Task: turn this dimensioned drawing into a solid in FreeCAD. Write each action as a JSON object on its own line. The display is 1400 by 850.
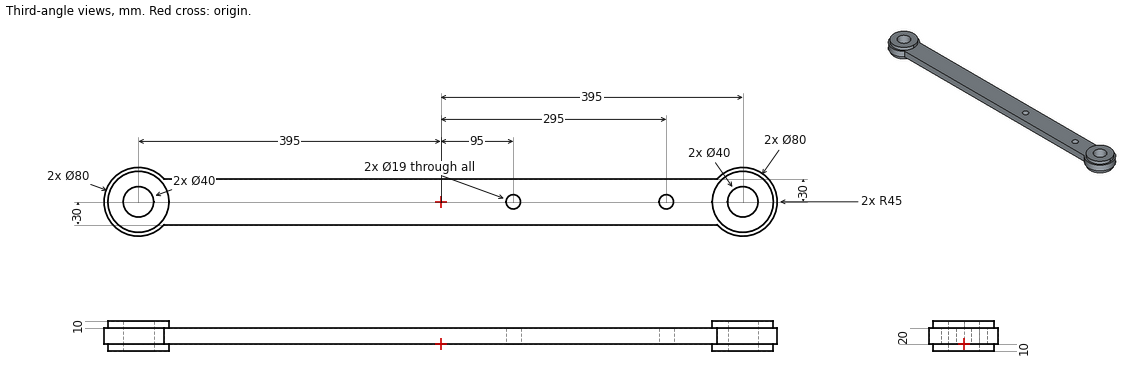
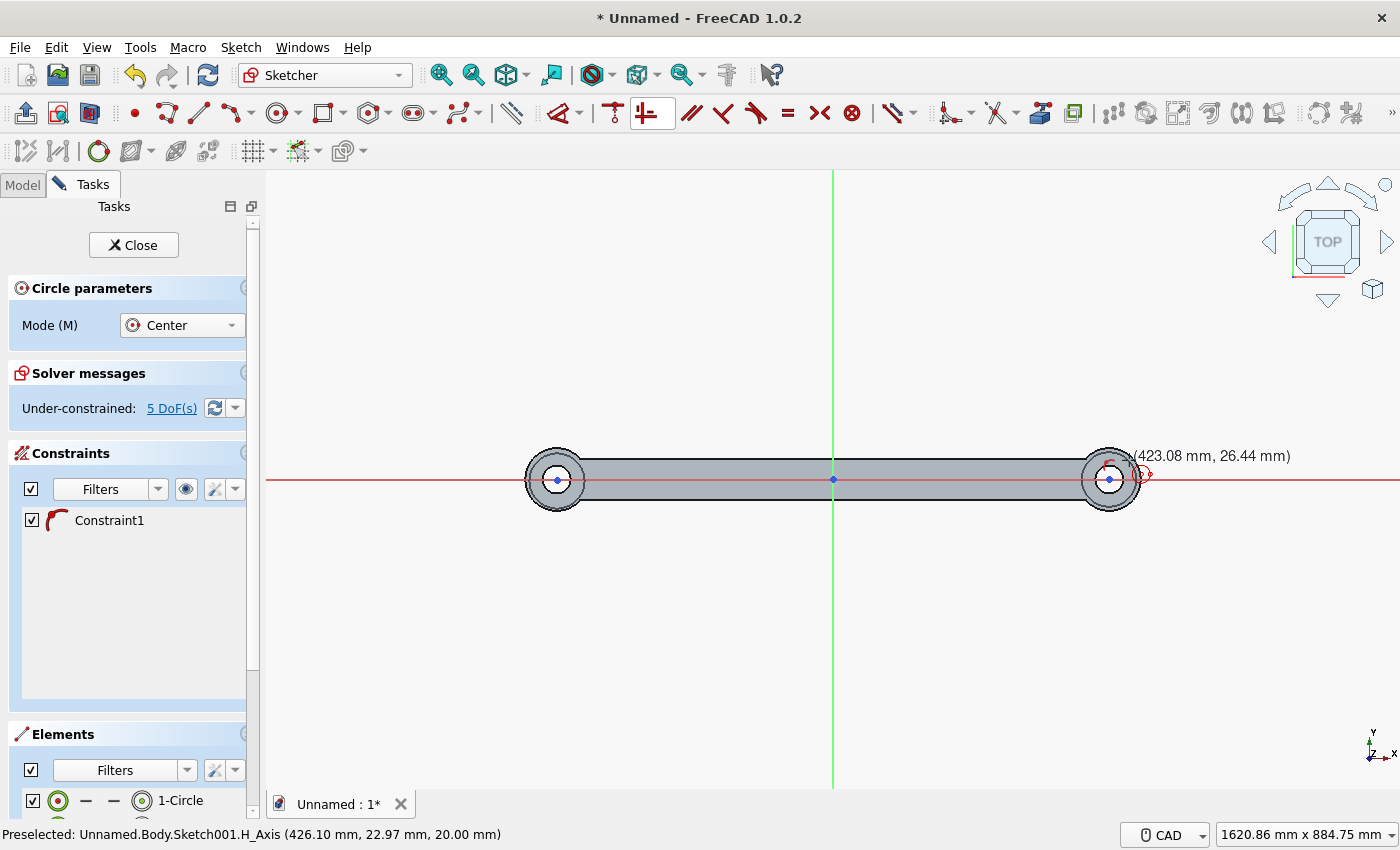
{"action": "scroll", "coordinate": [557, 480], "scroll_direction": "up", "scroll_amount": 3}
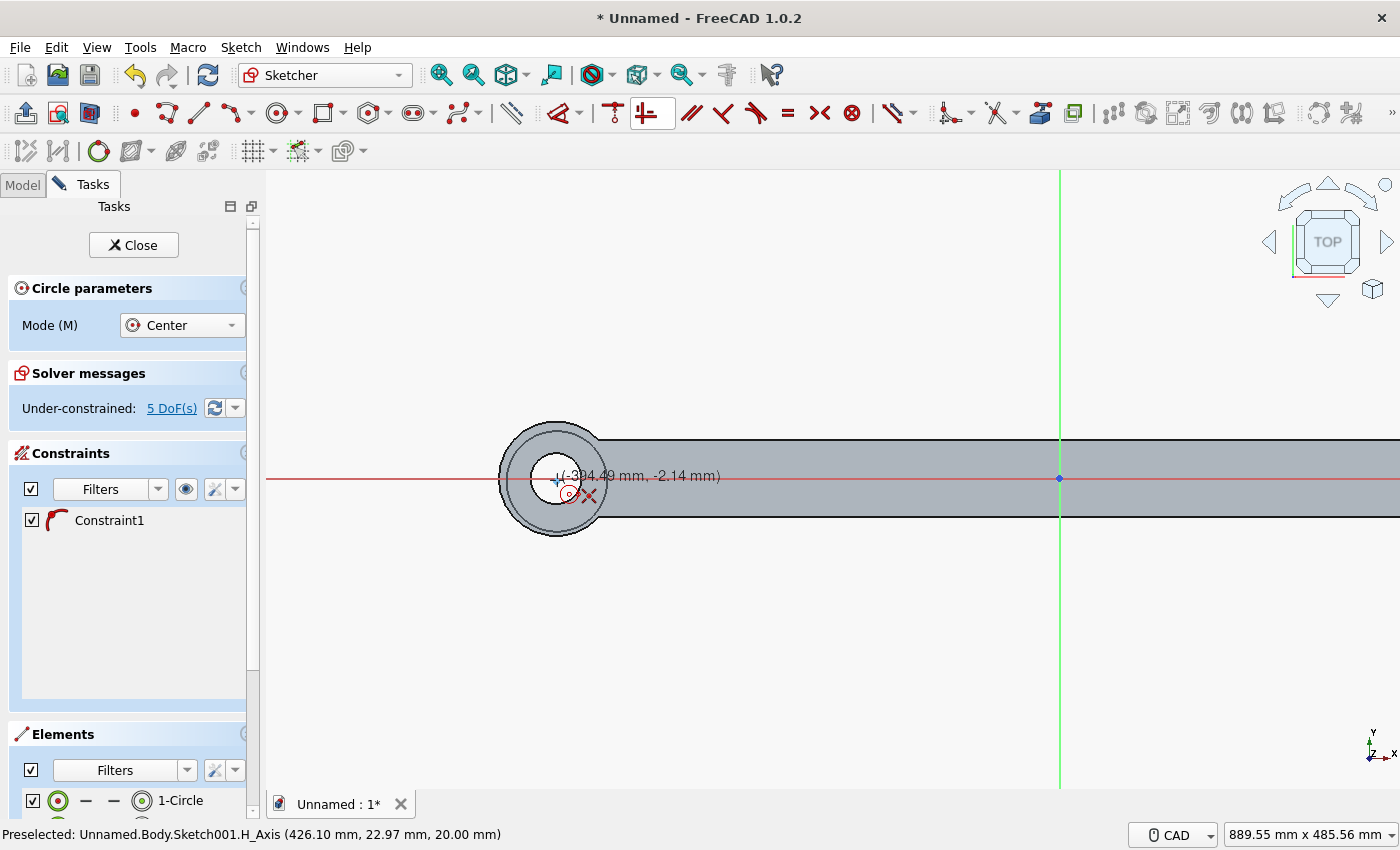
{"action": "left_click", "coordinate": [557, 481]}
{"action": "left_click", "coordinate": [574, 461]}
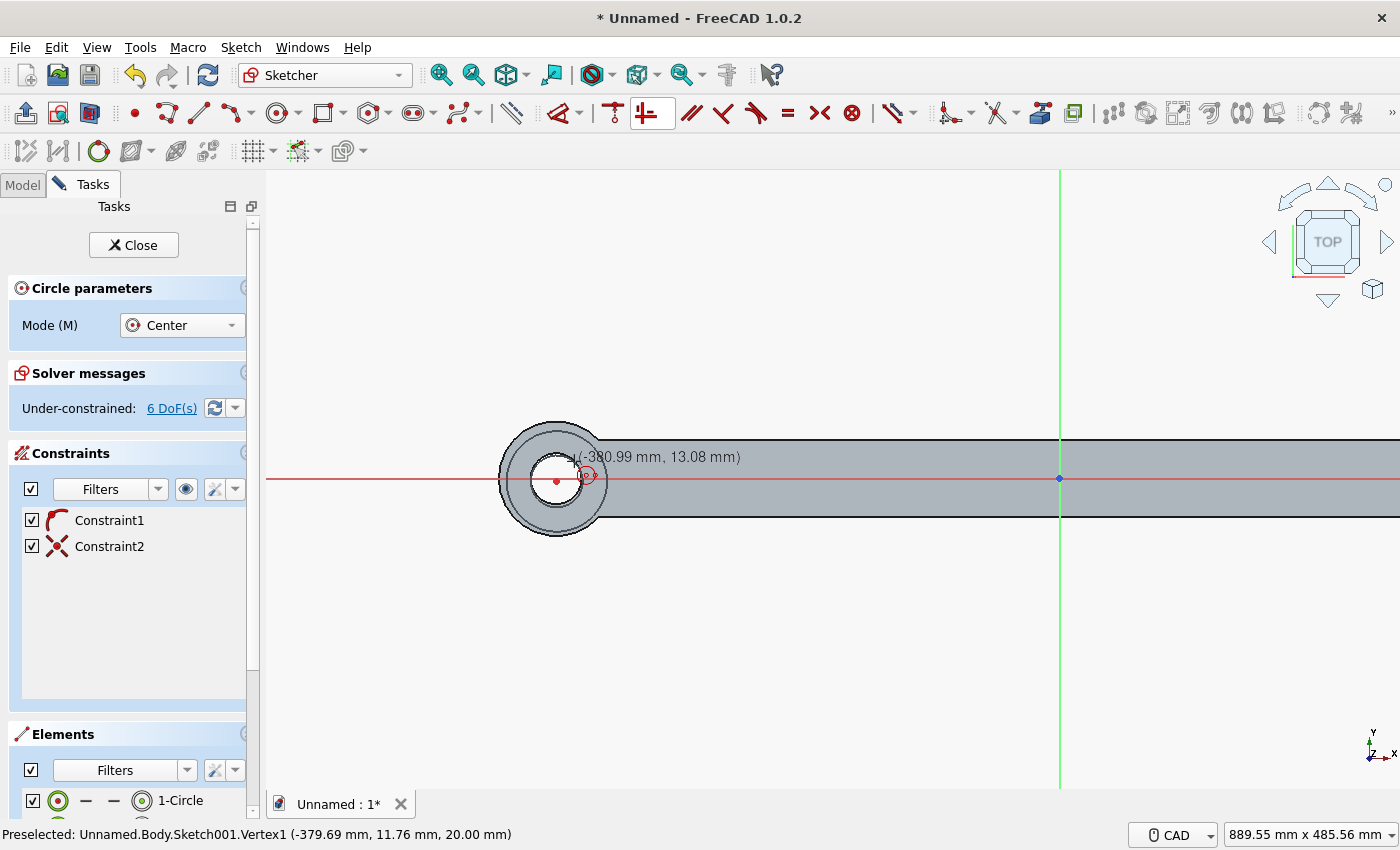
{"action": "scroll", "coordinate": [405, 481], "scroll_direction": "down", "scroll_amount": 3}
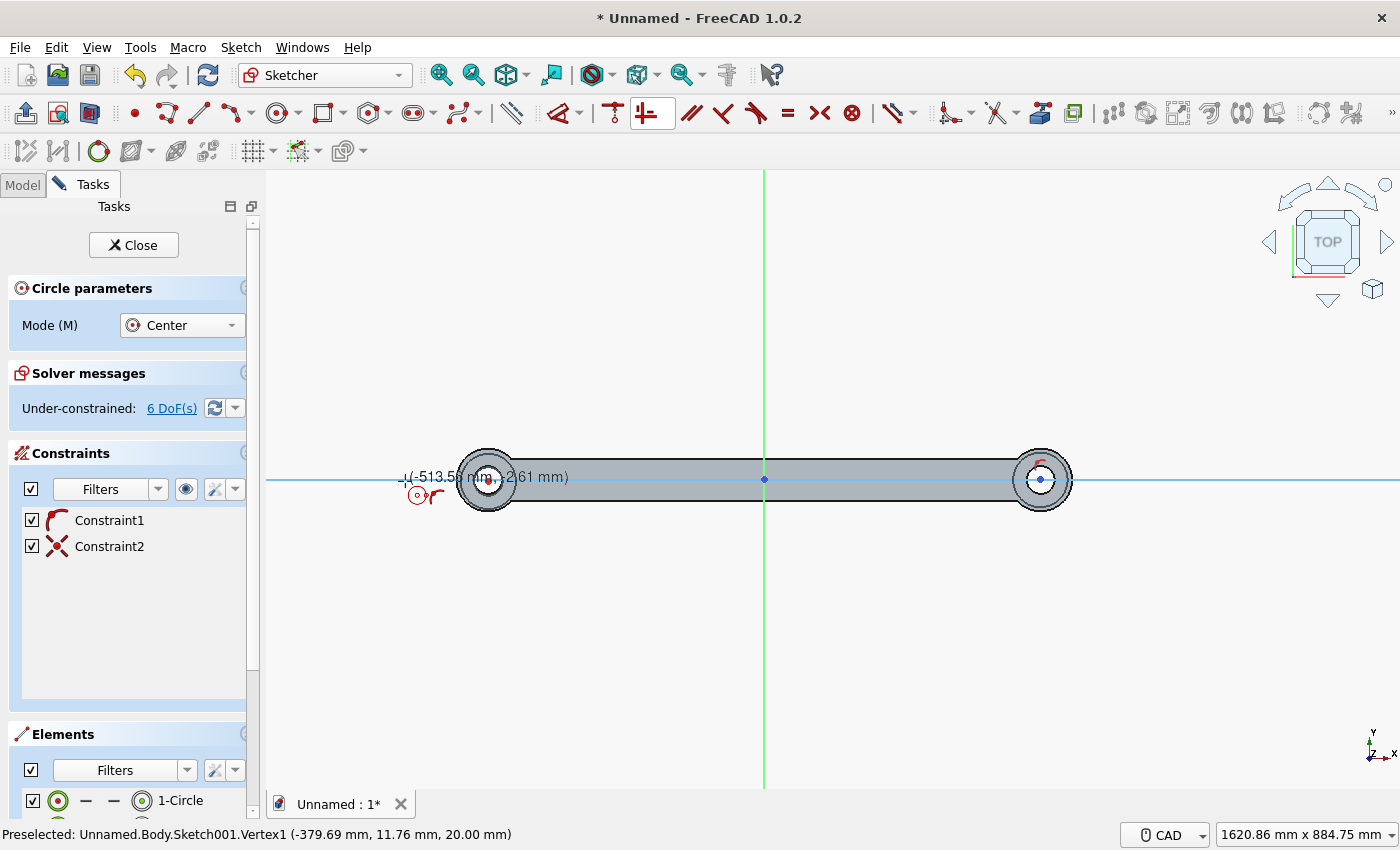
{"action": "scroll", "coordinate": [1041, 480], "scroll_direction": "up", "scroll_amount": 3}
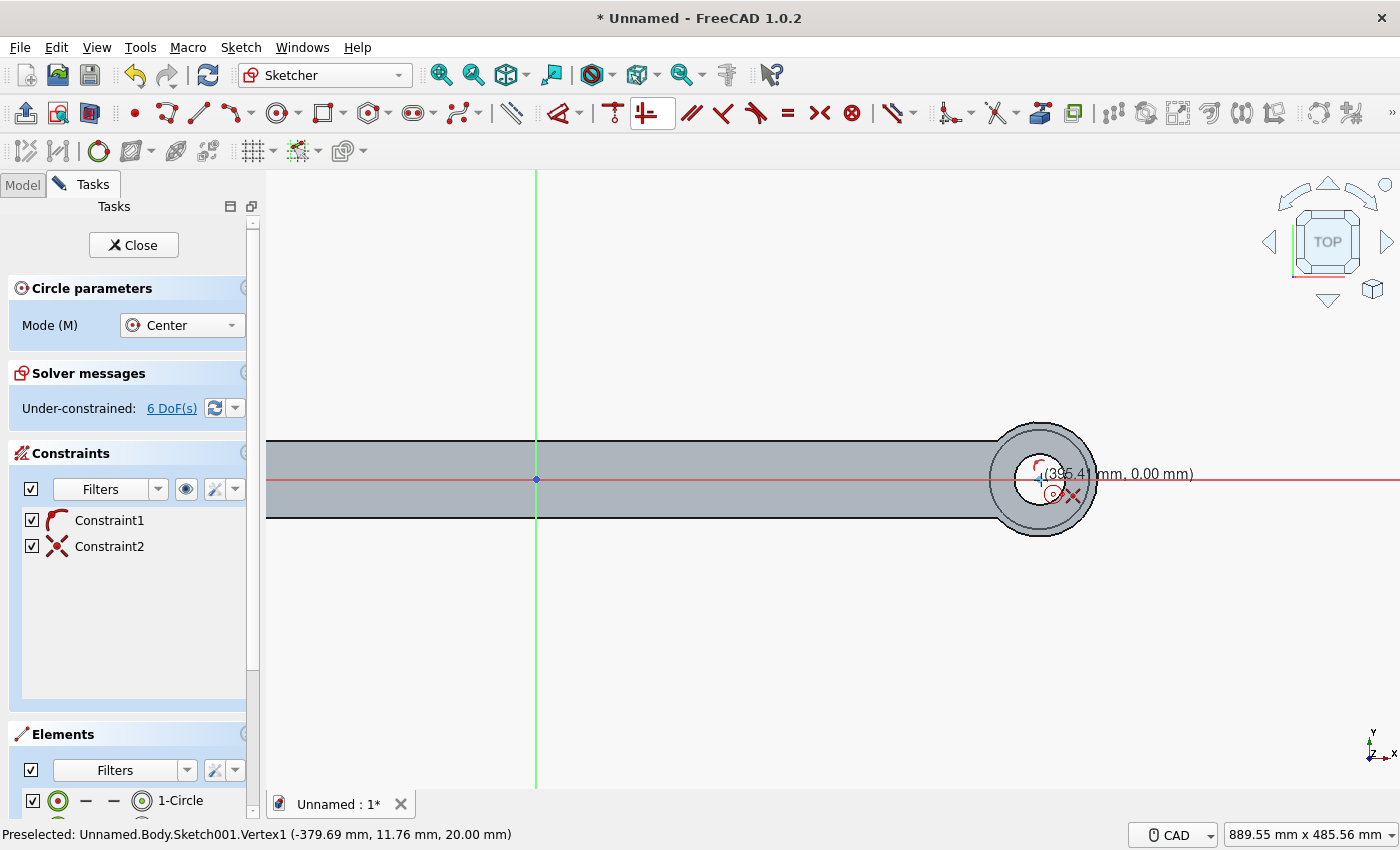
{"action": "left_click", "coordinate": [1039, 480]}
{"action": "left_click", "coordinate": [1058, 461]}
{"action": "key", "text": "Escape"}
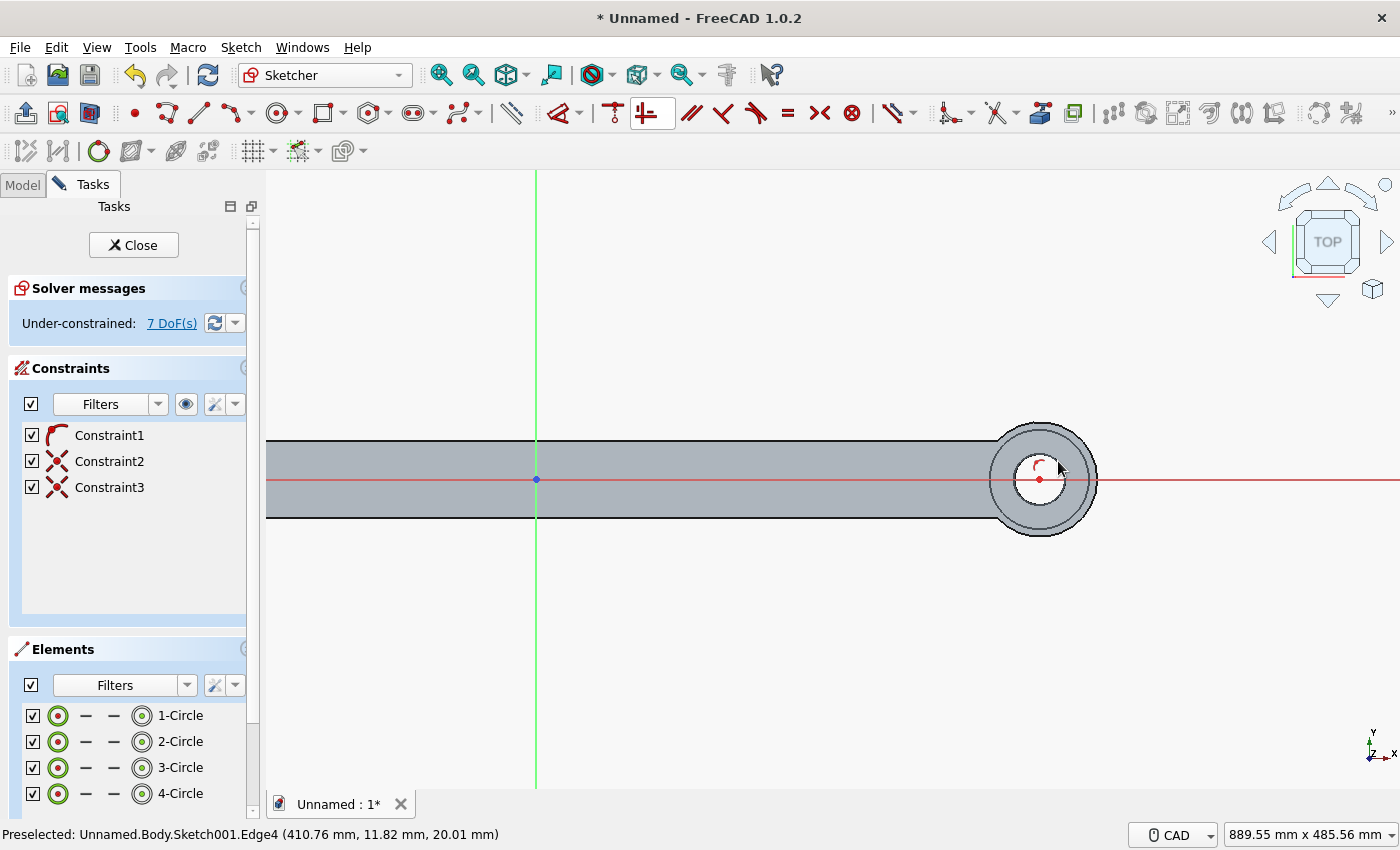
{"action": "scroll", "coordinate": [1042, 479], "scroll_direction": "down", "scroll_amount": 3}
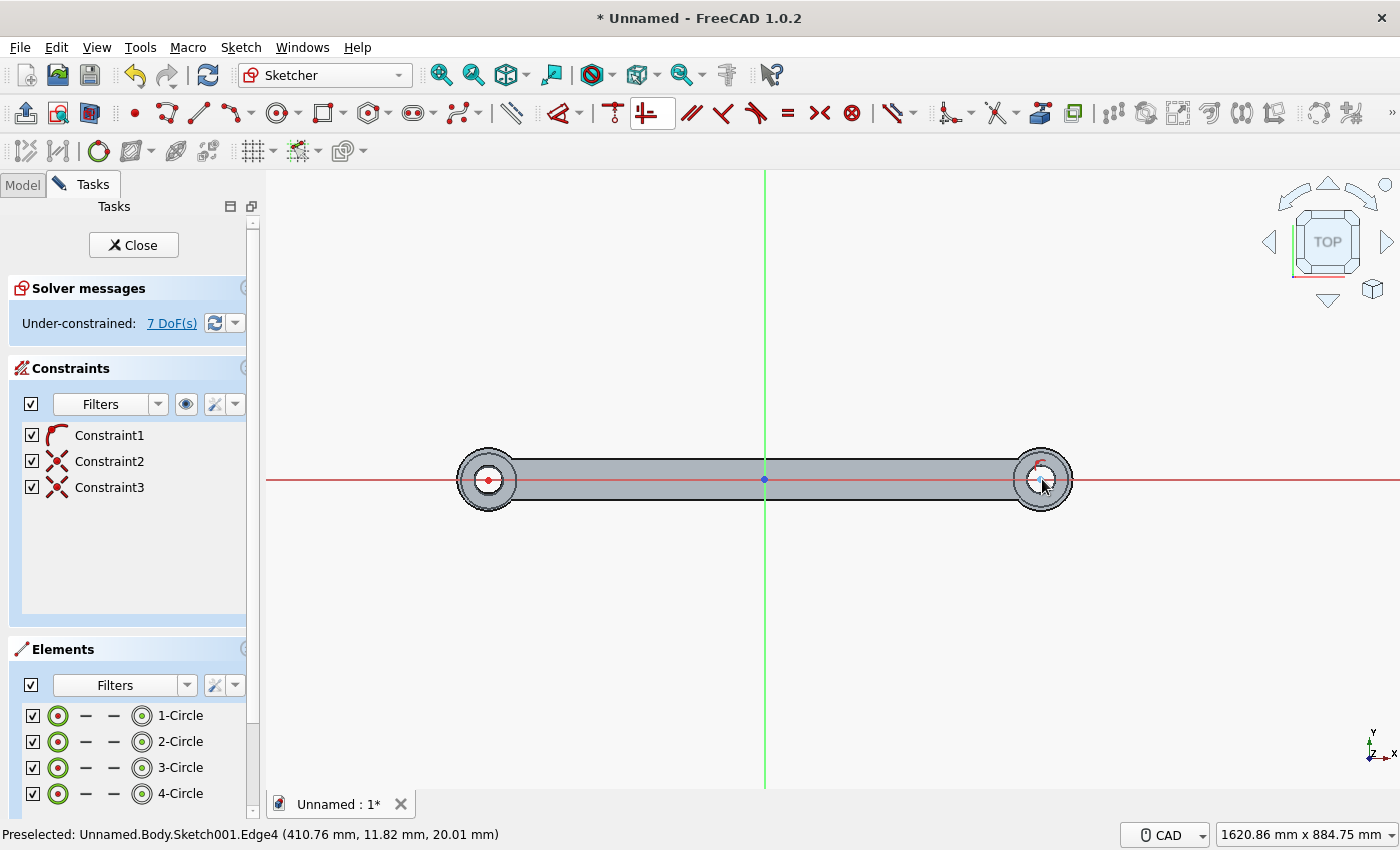
{"action": "left_click", "coordinate": [508, 461]}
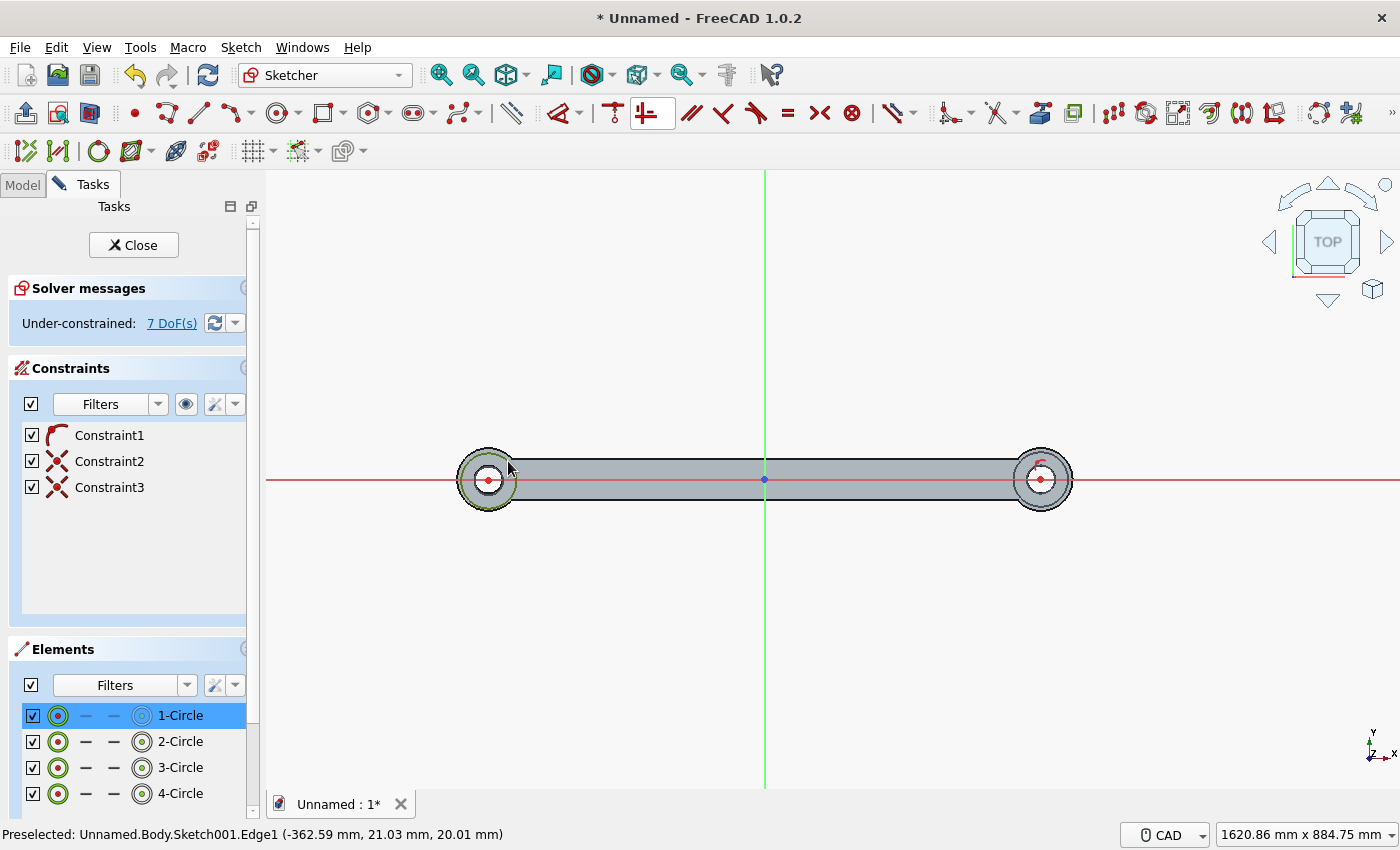
{"action": "left_click", "coordinate": [1060, 460]}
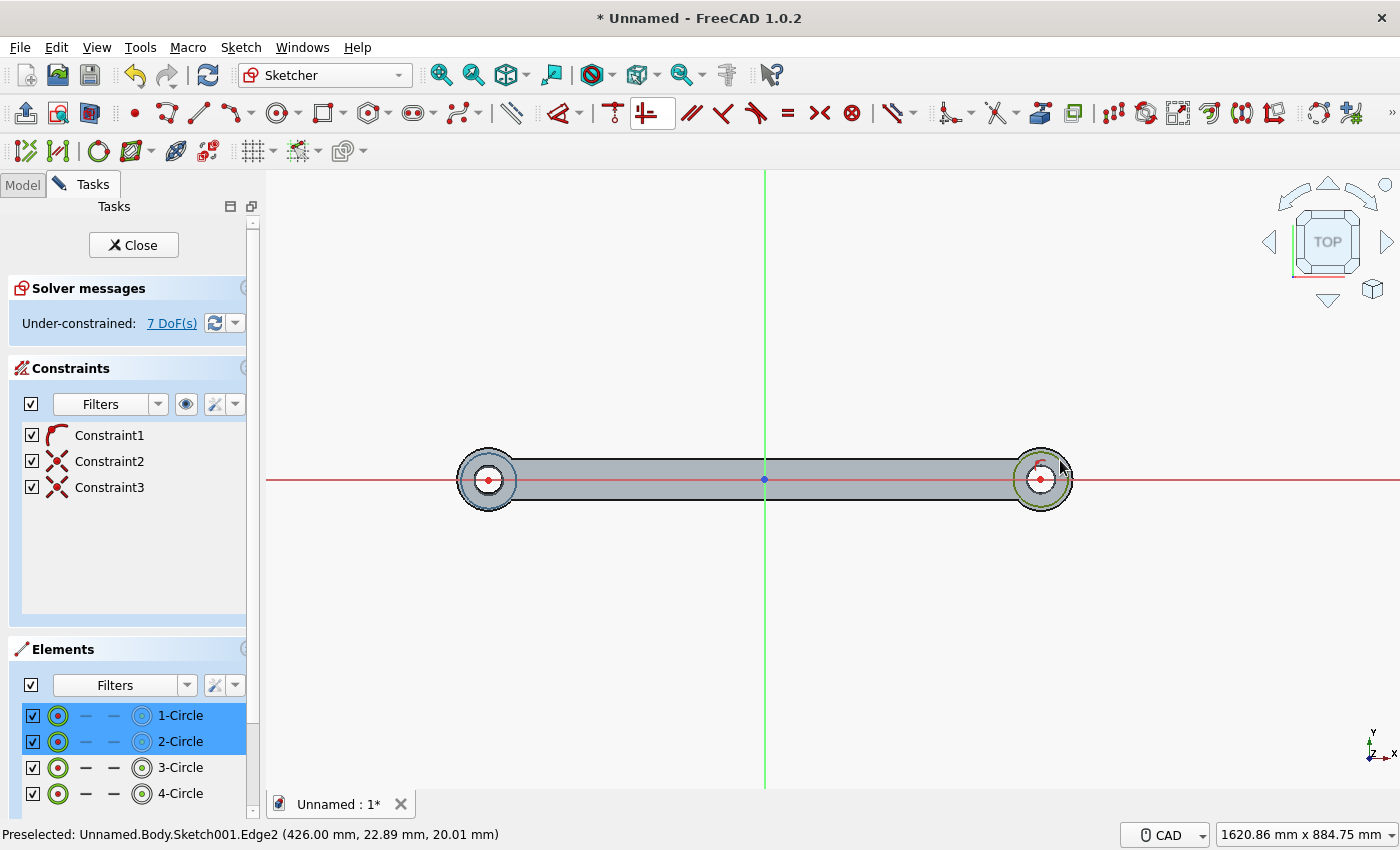
{"action": "left_click", "coordinate": [788, 114]}